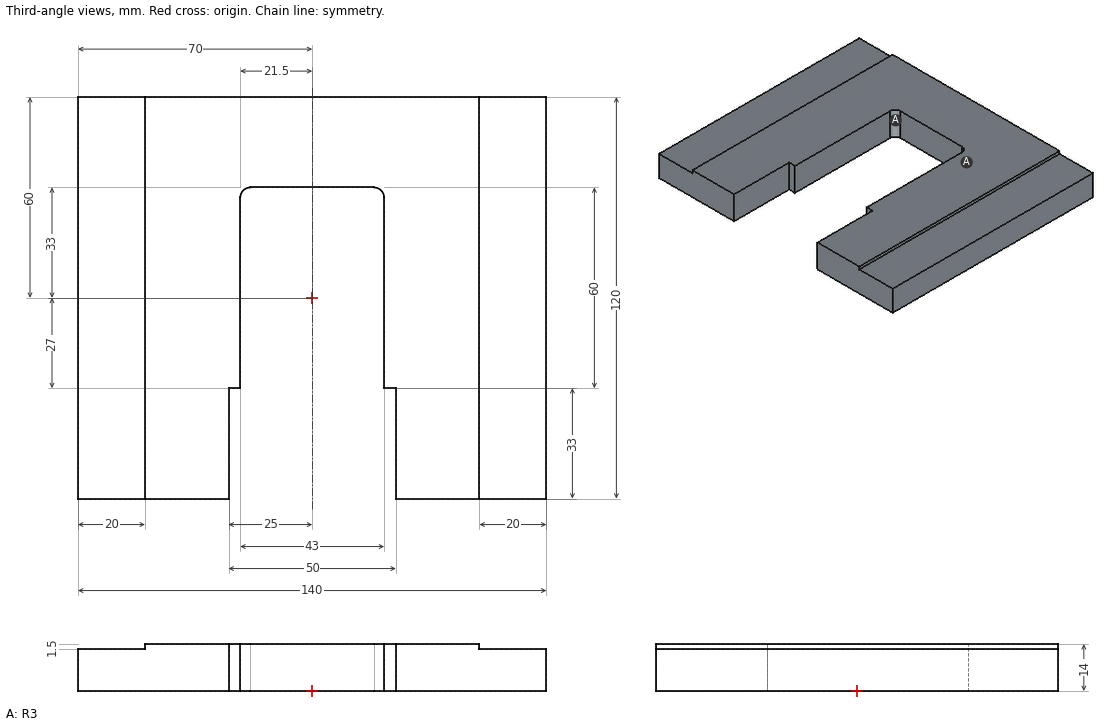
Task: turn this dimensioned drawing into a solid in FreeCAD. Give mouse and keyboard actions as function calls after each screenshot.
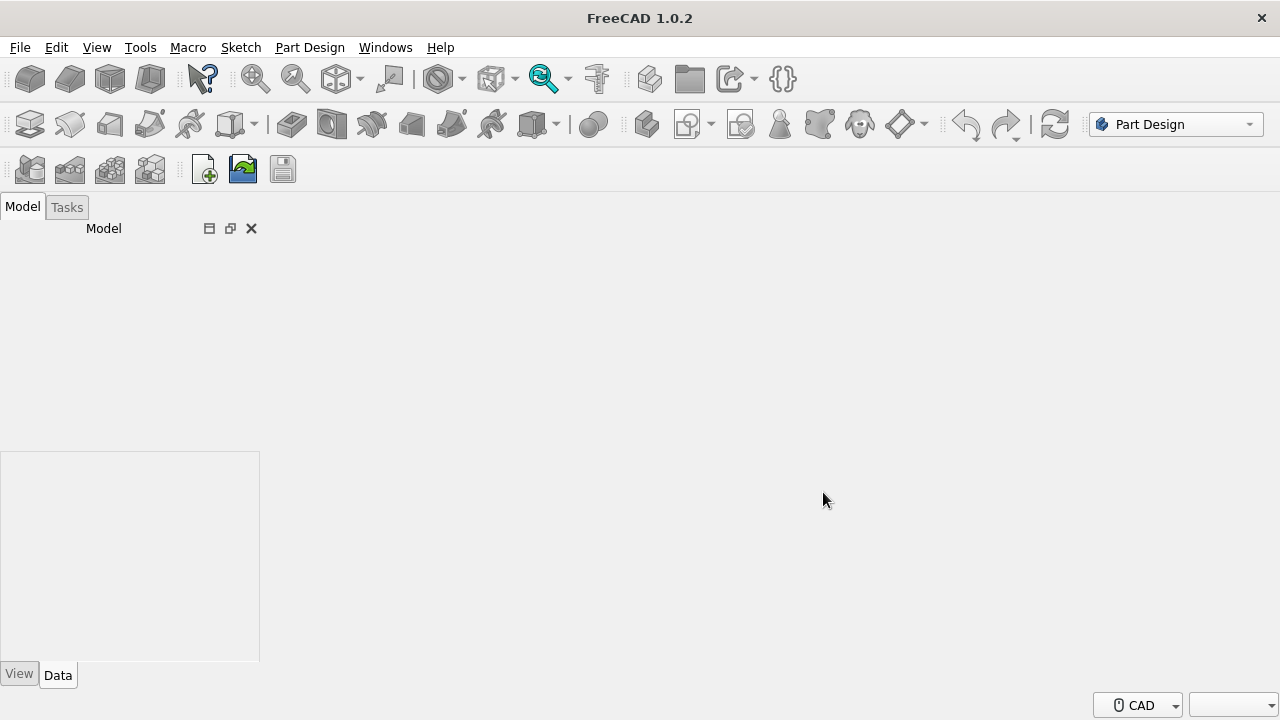
click(204, 170)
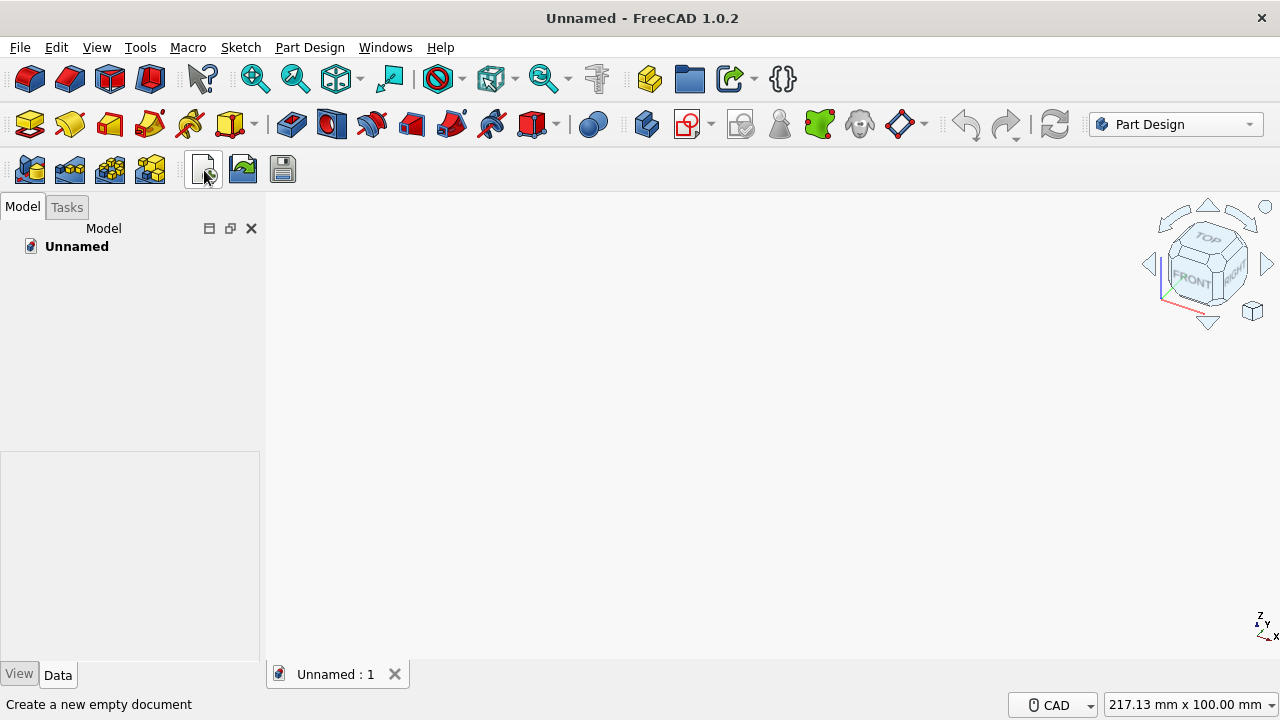
click(688, 124)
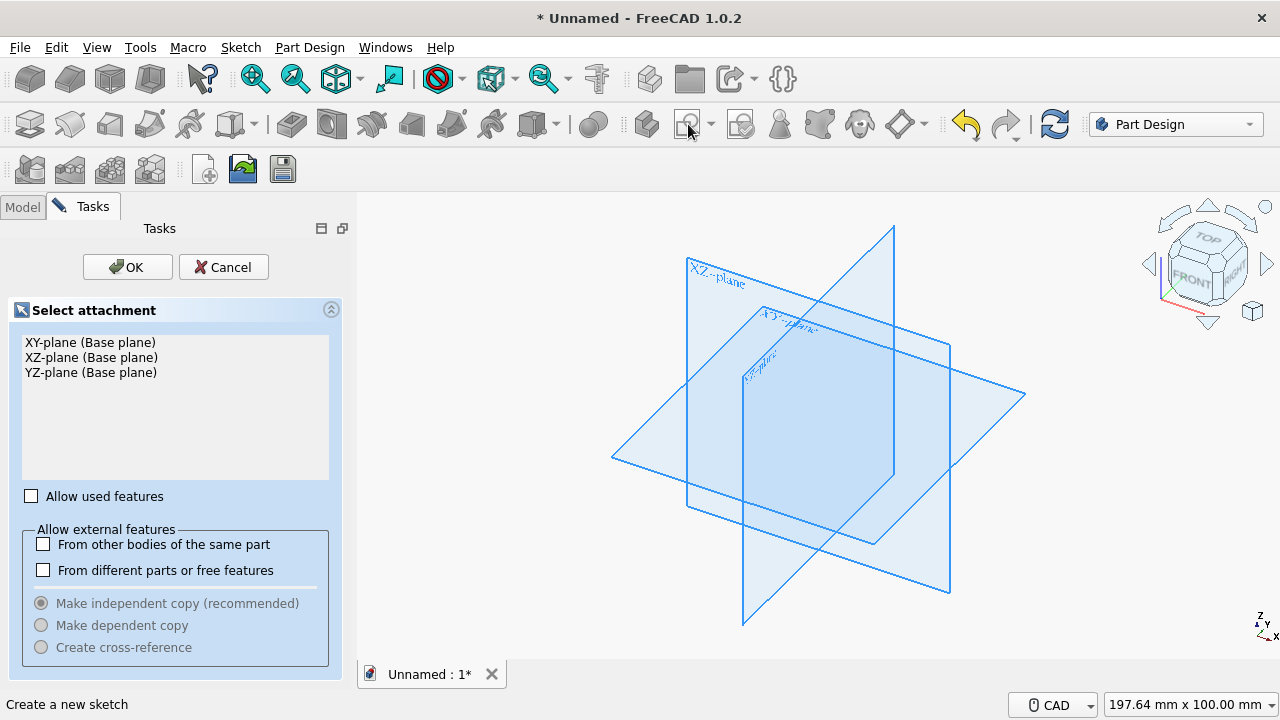
click(82, 342)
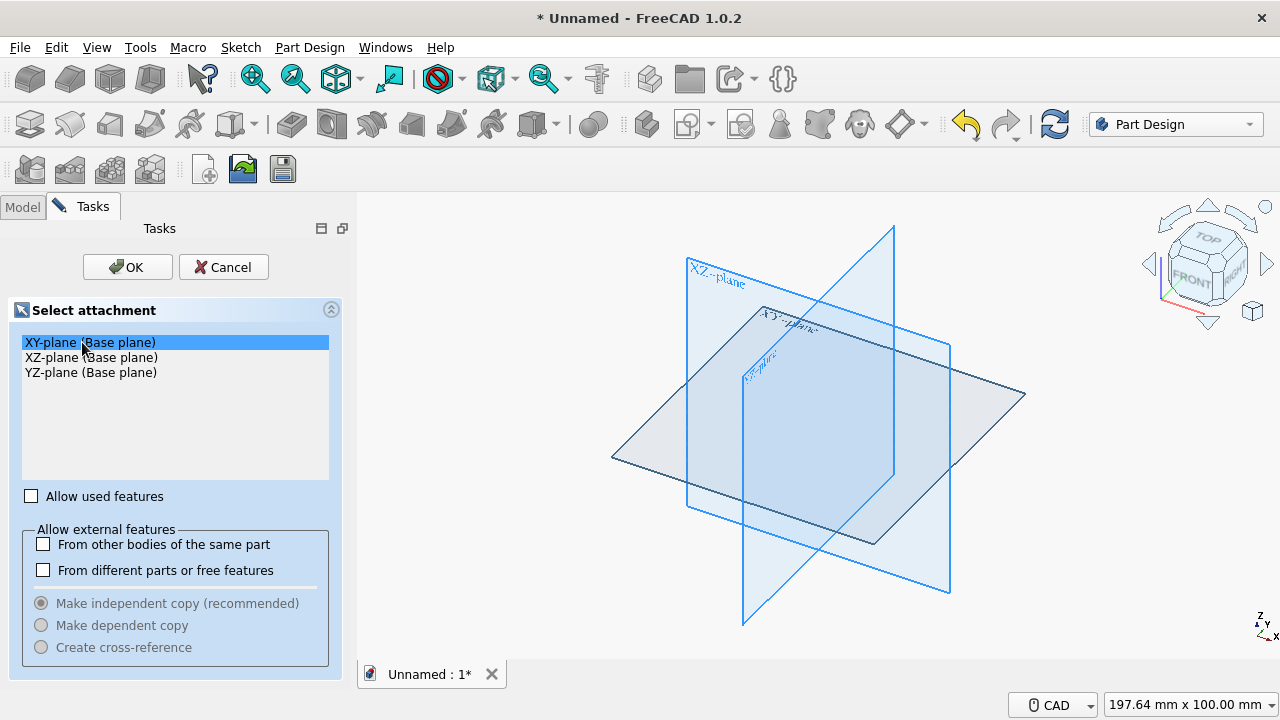
click(128, 267)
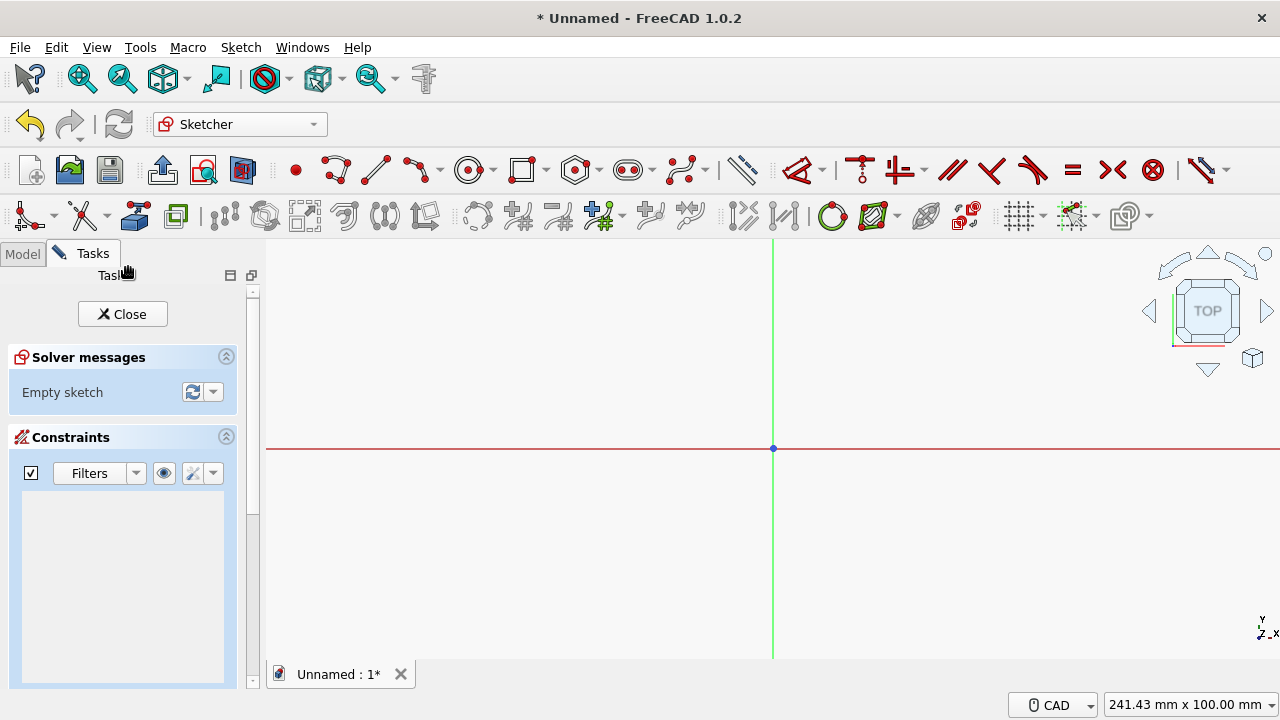
scroll(621, 449, down, 3)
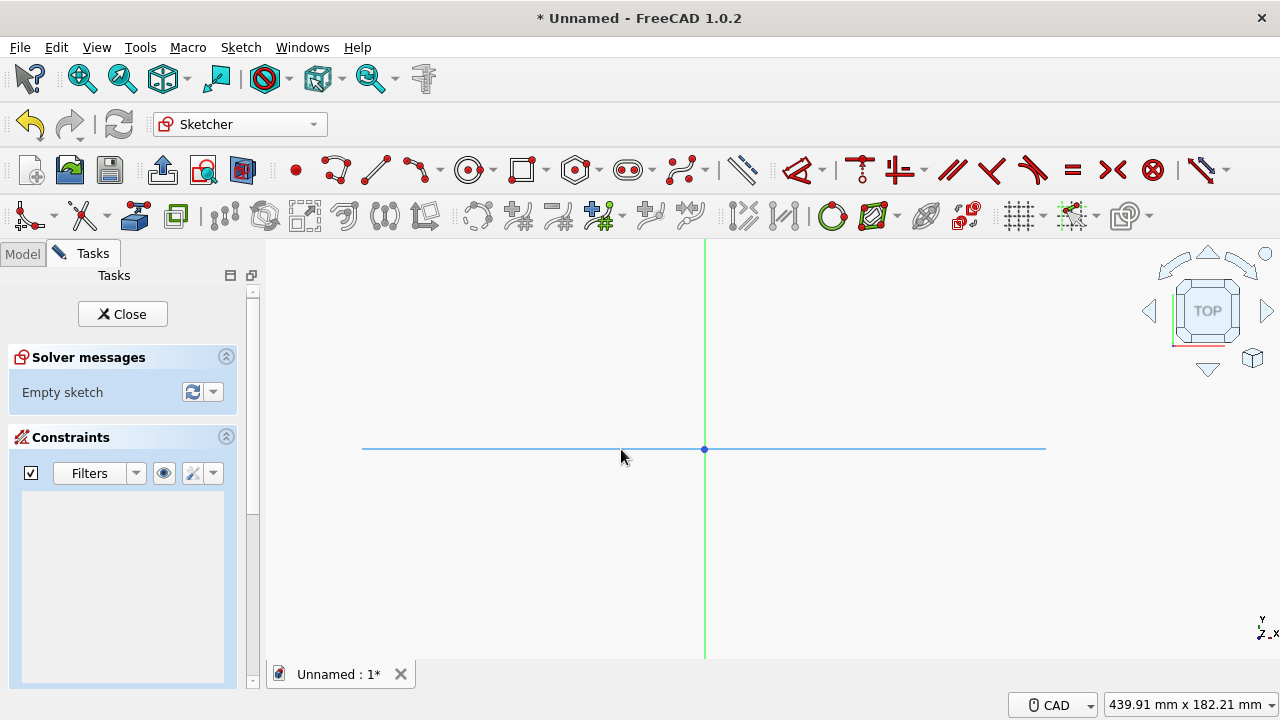
click(548, 170)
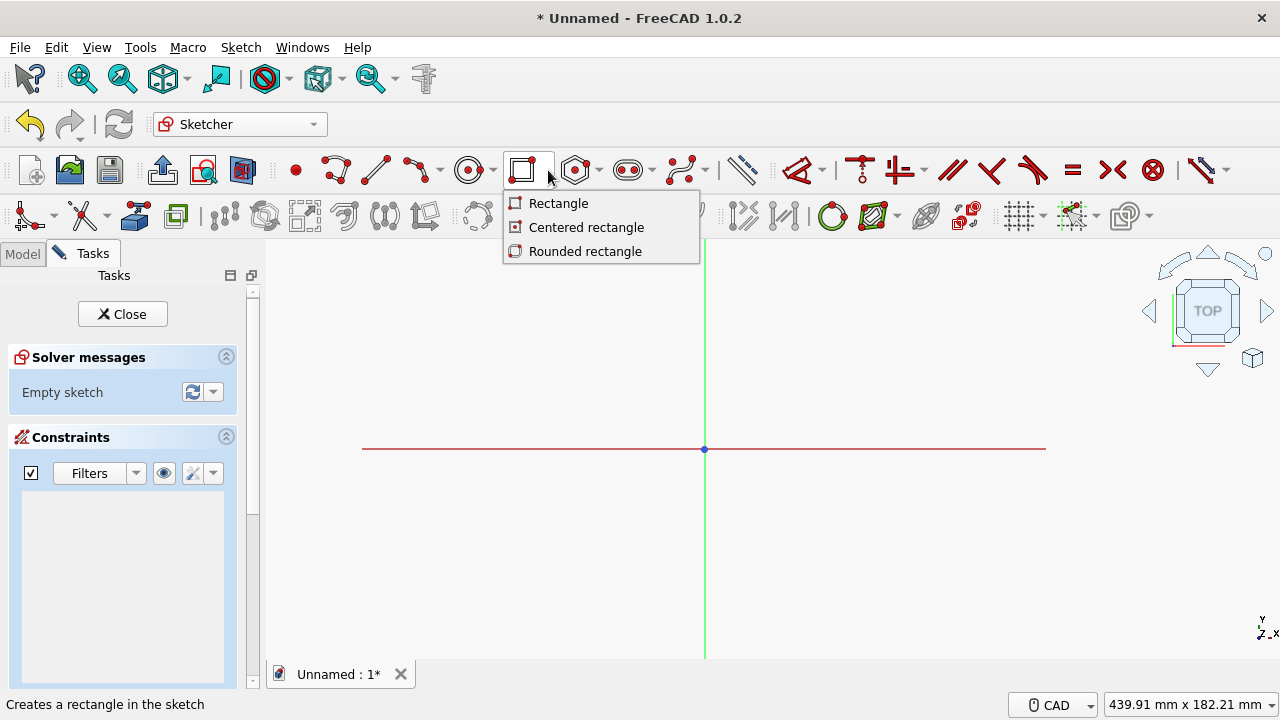
click(602, 227)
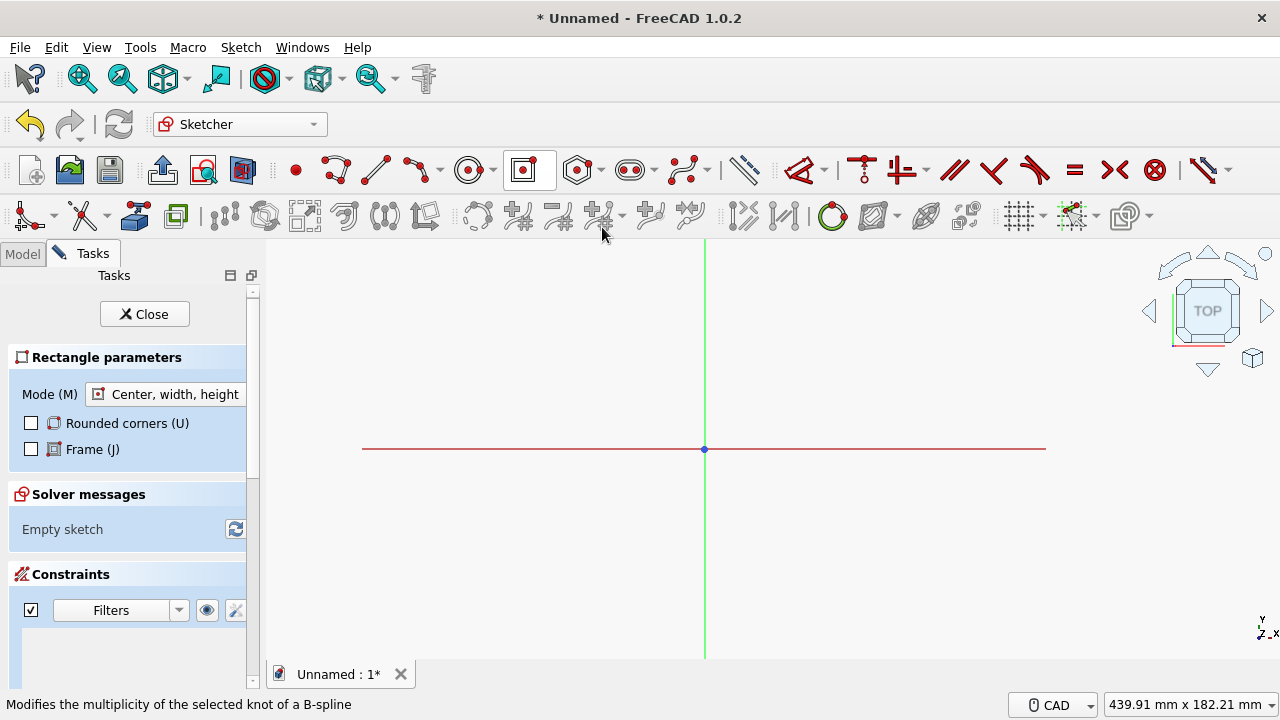
click(705, 449)
move(866, 311)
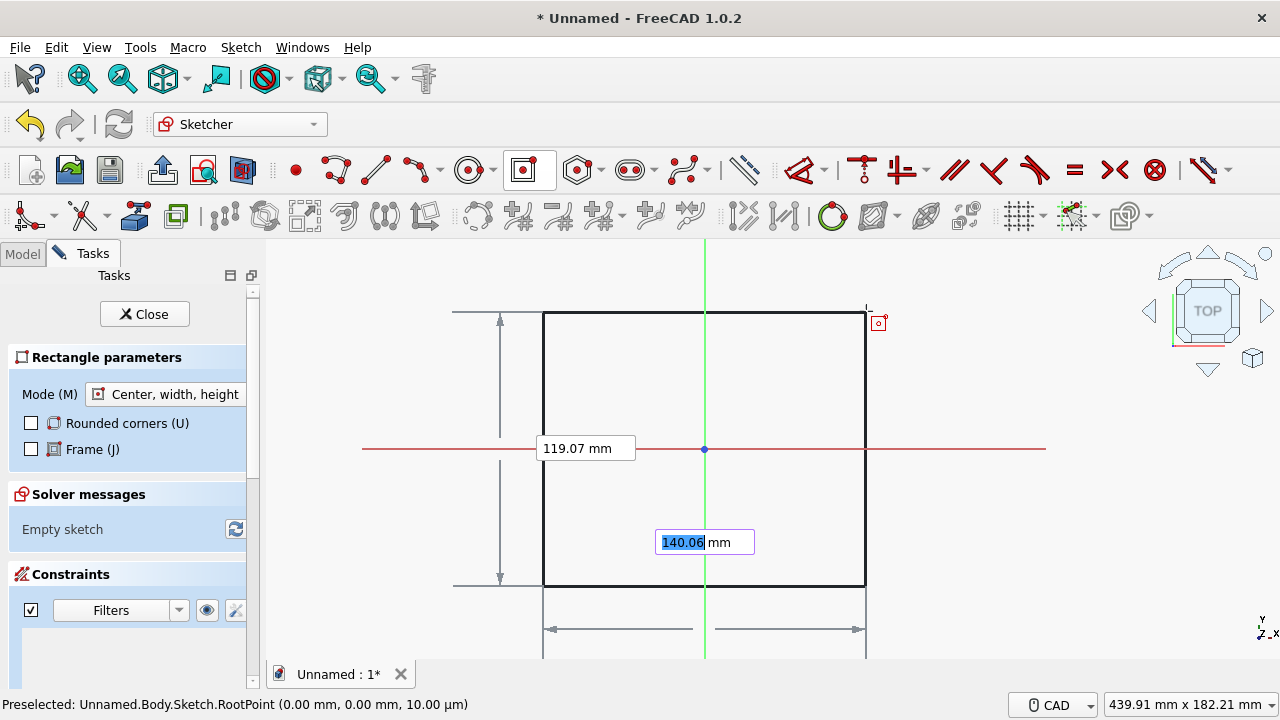
text(140)
key(Tab)
text(120)
key(Return)
key(Escape)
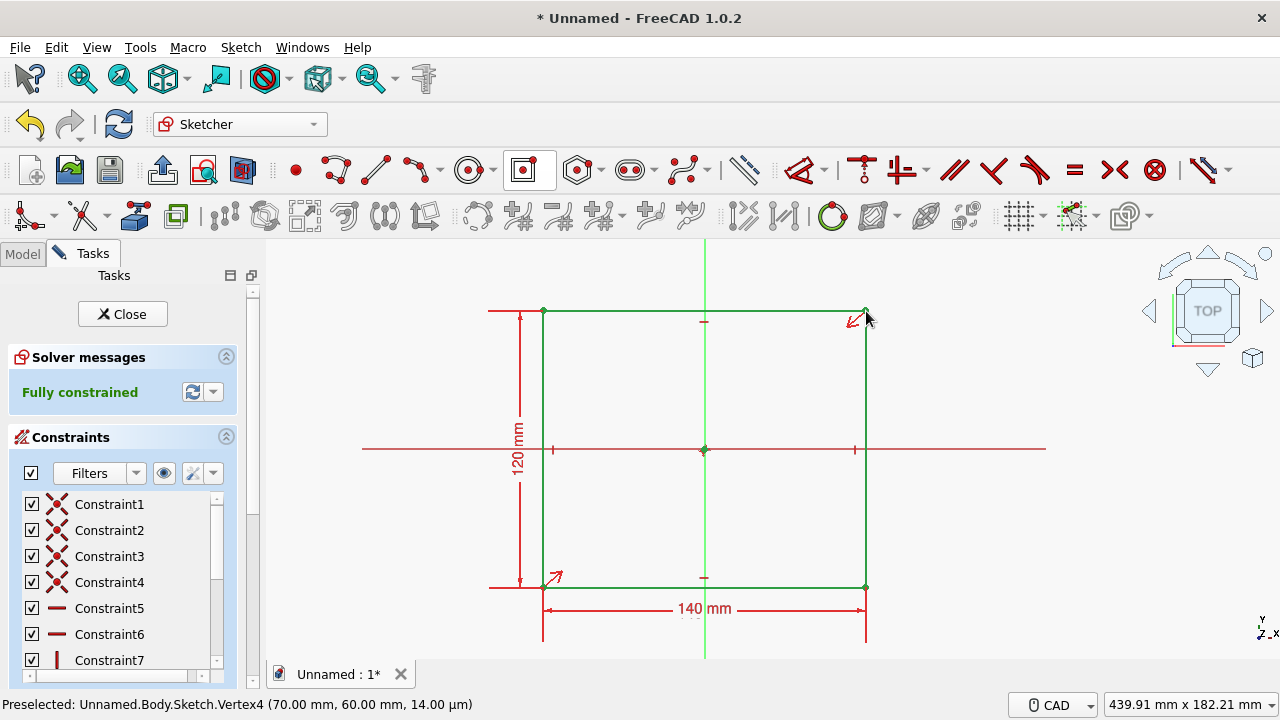
click(123, 314)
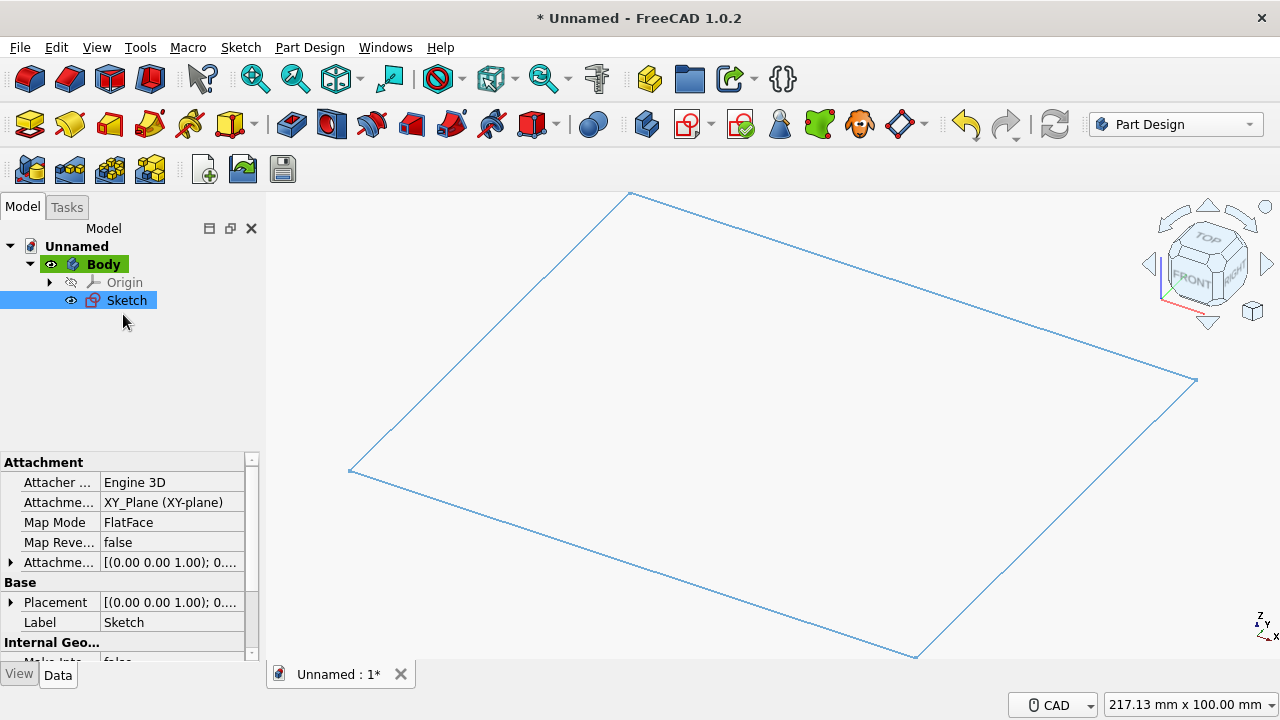
click(30, 124)